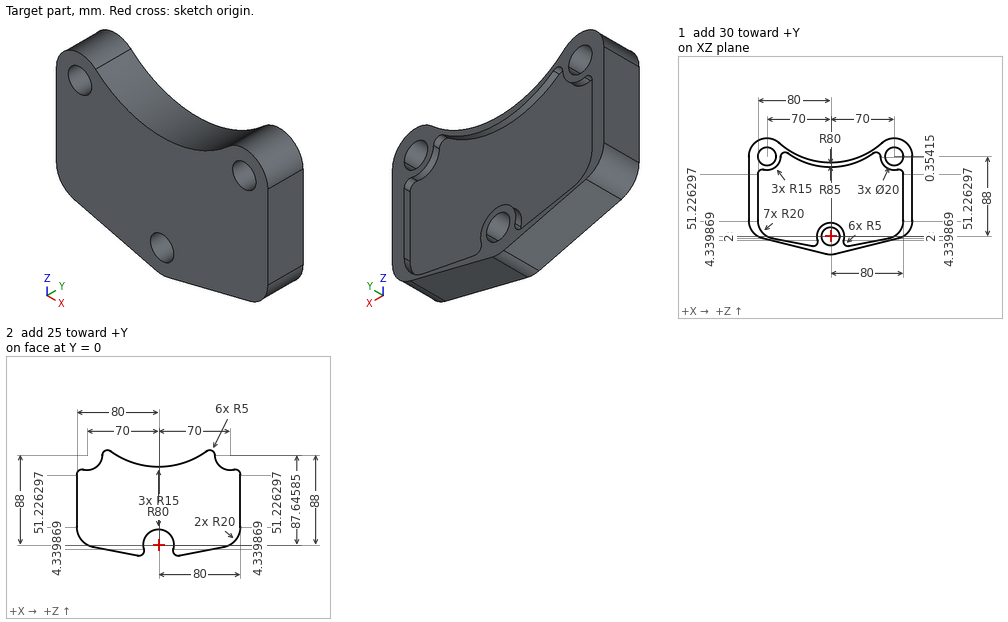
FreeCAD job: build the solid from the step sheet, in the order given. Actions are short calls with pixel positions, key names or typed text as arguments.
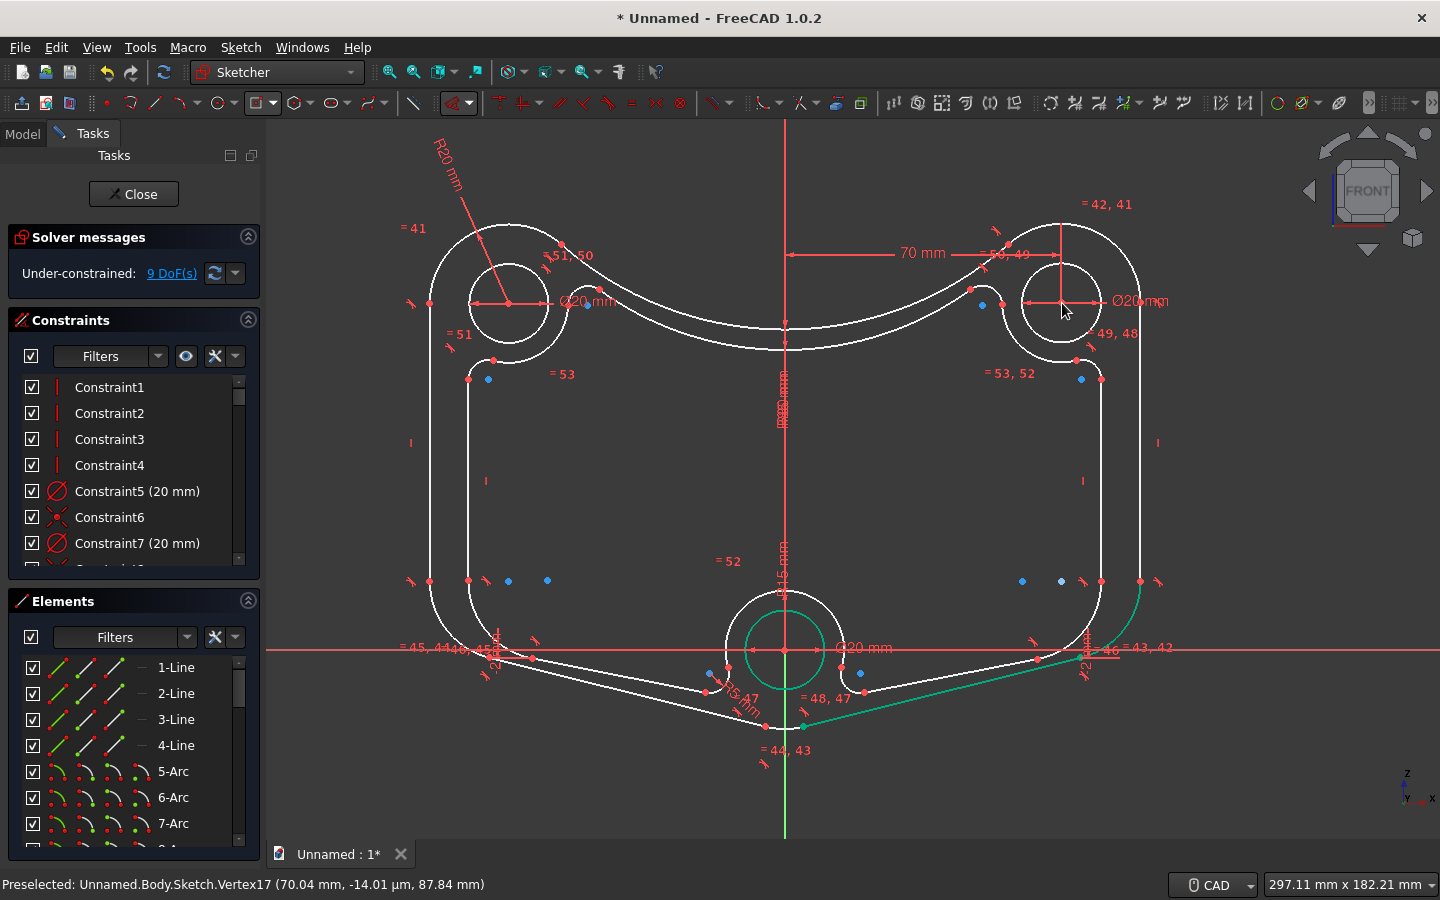
click(1061, 303)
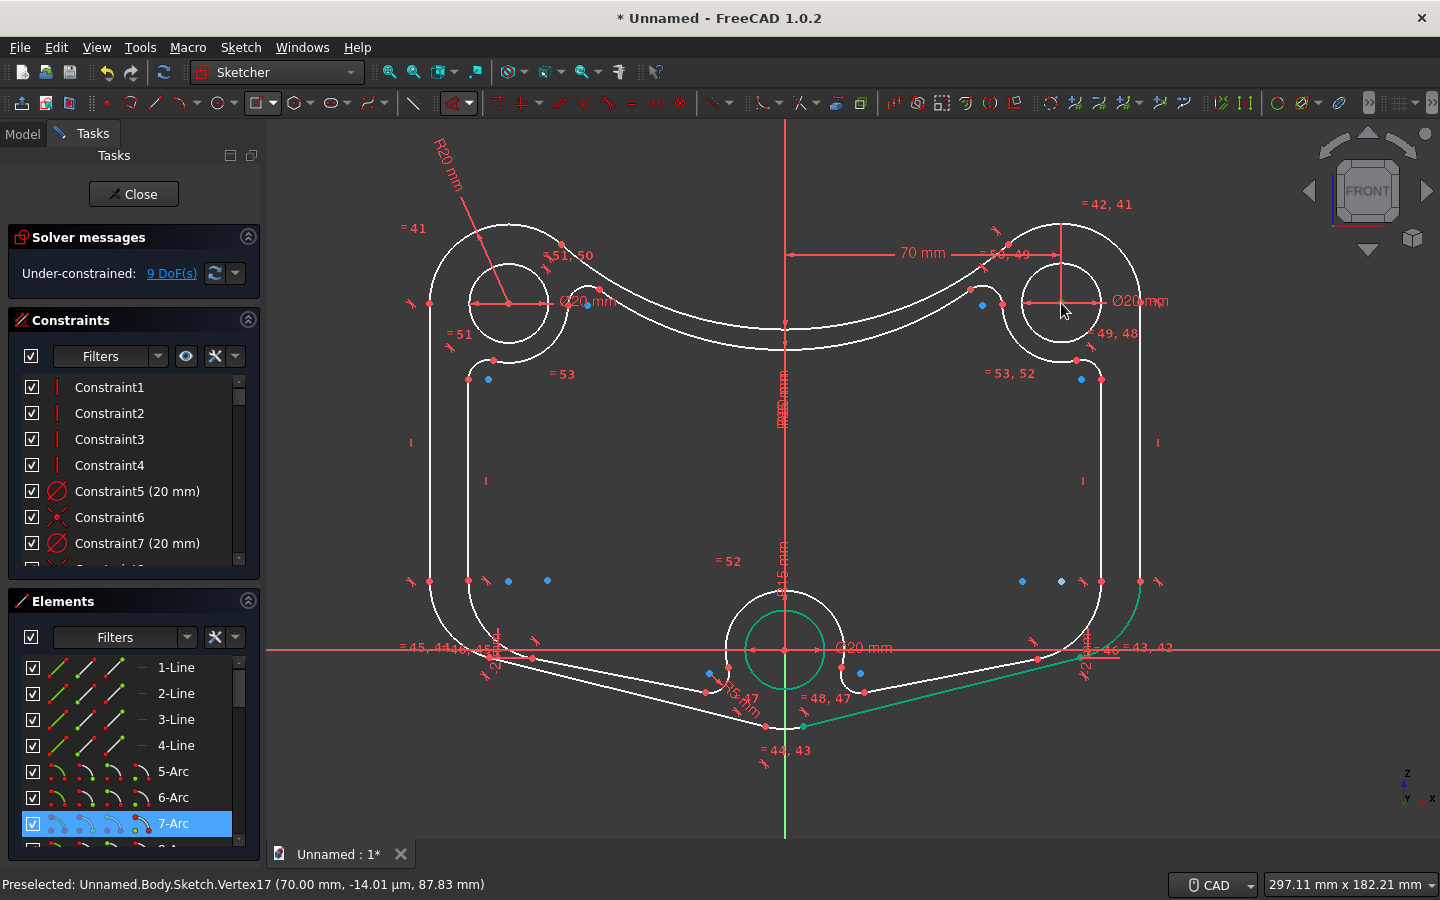
click(472, 104)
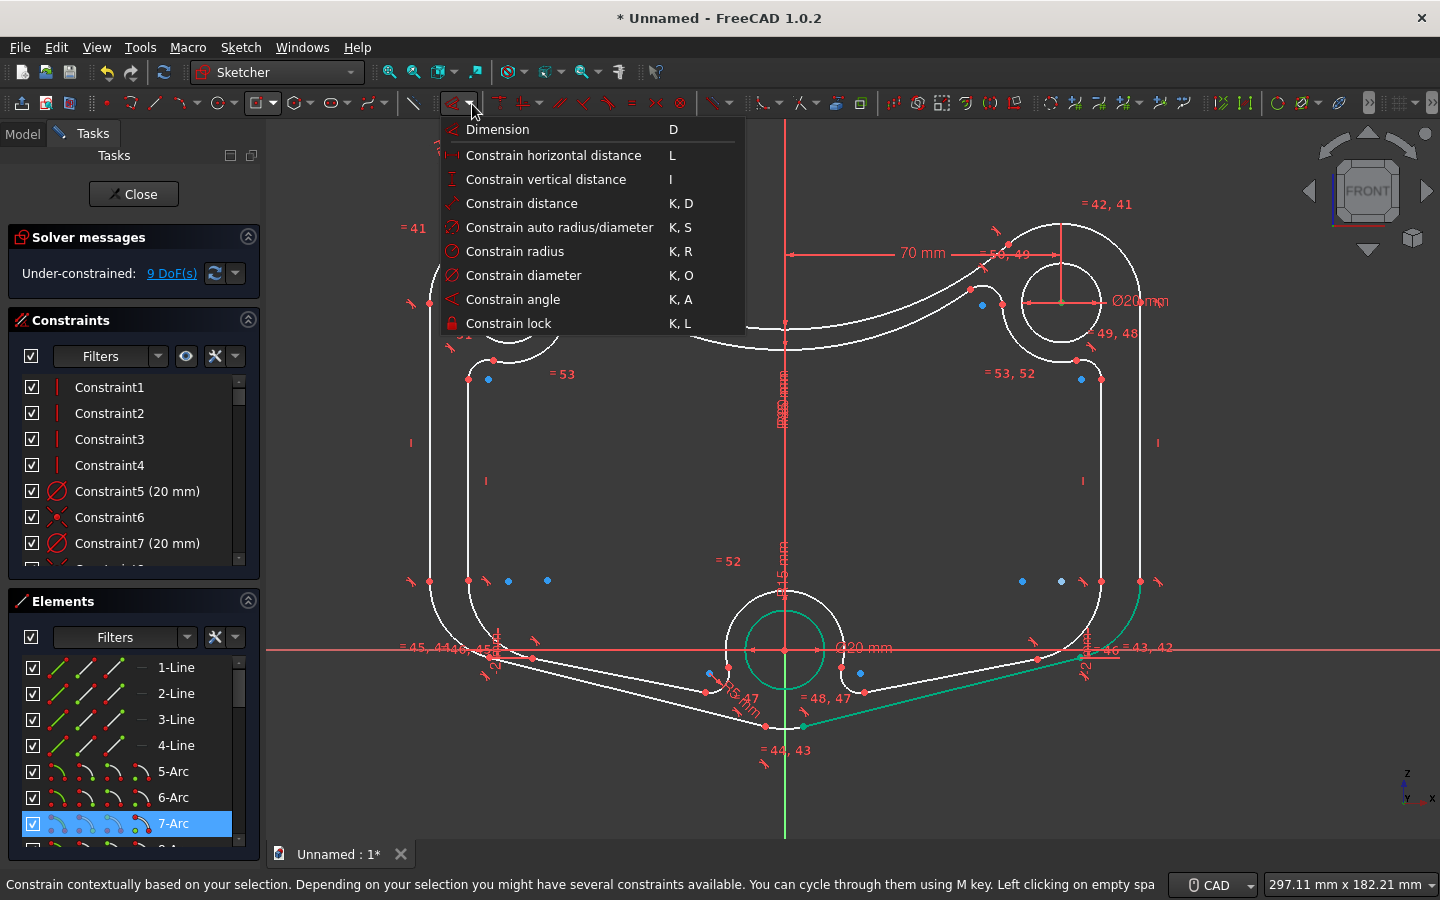
click(593, 179)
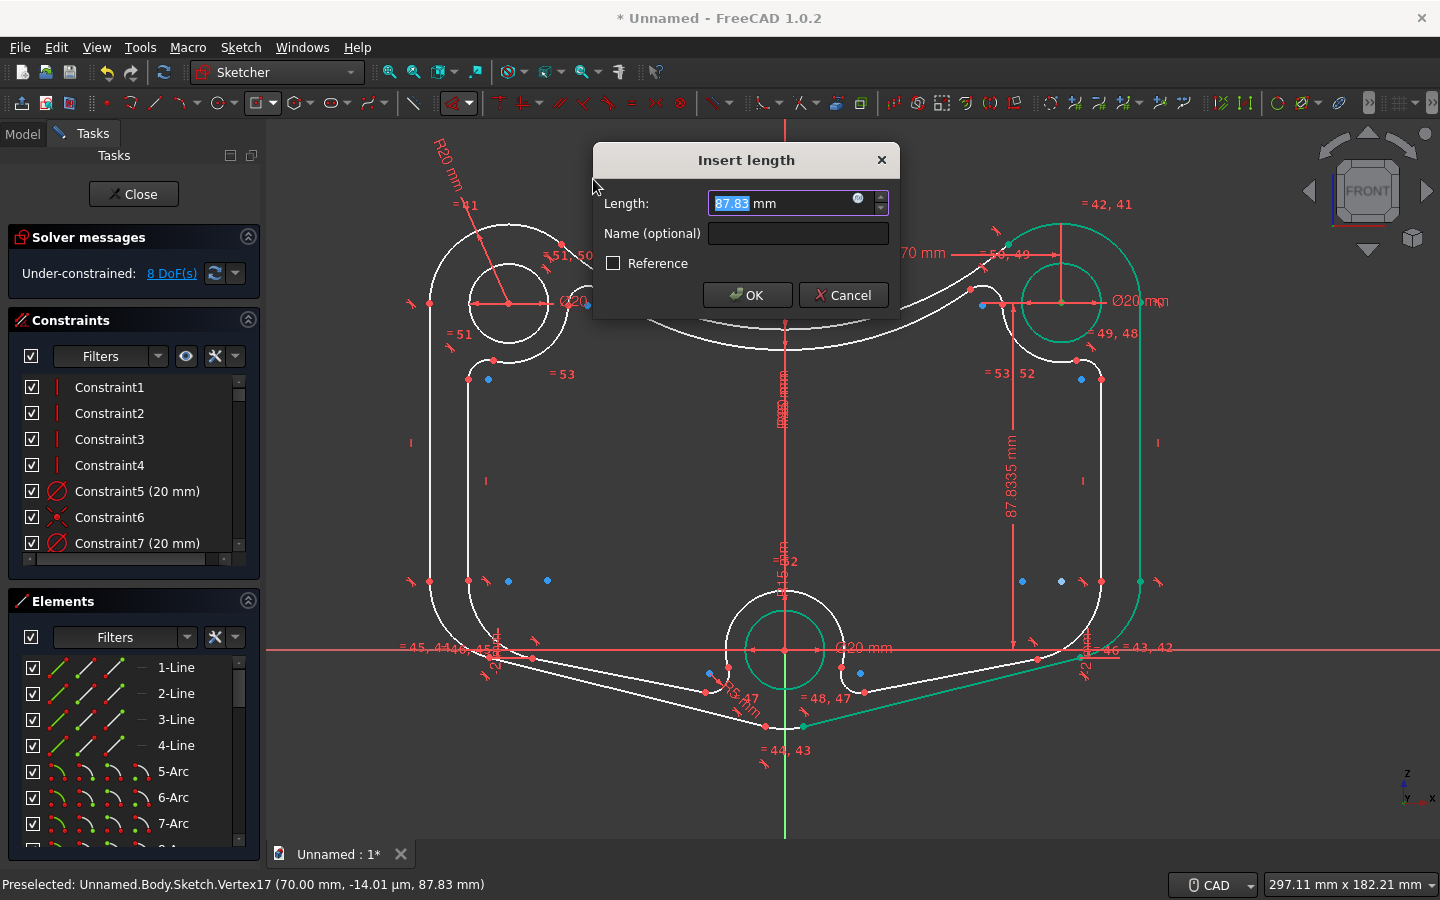
text(88)
key(Return)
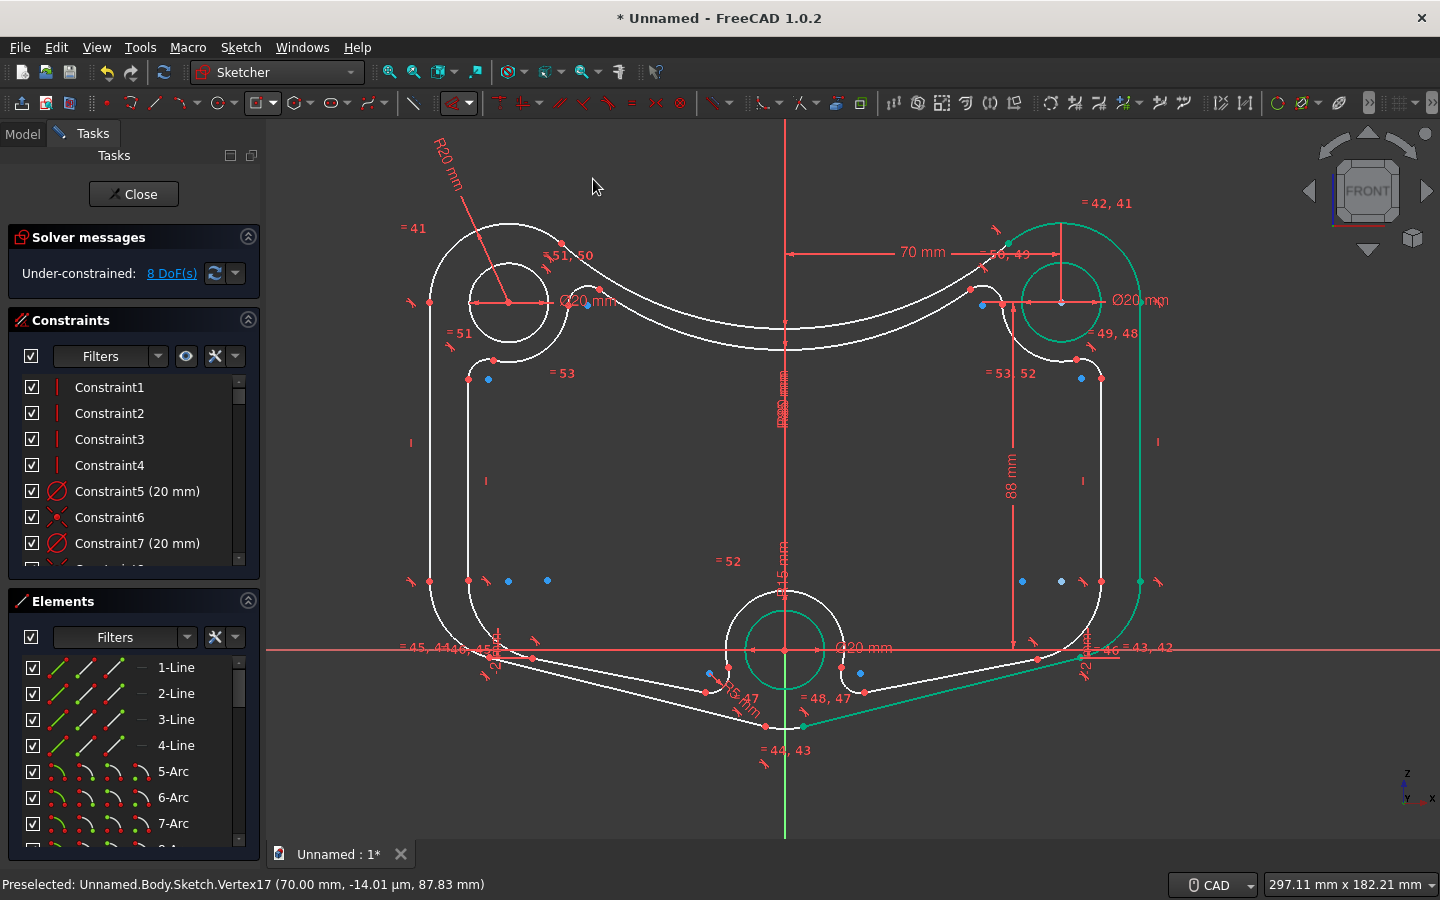
click(509, 303)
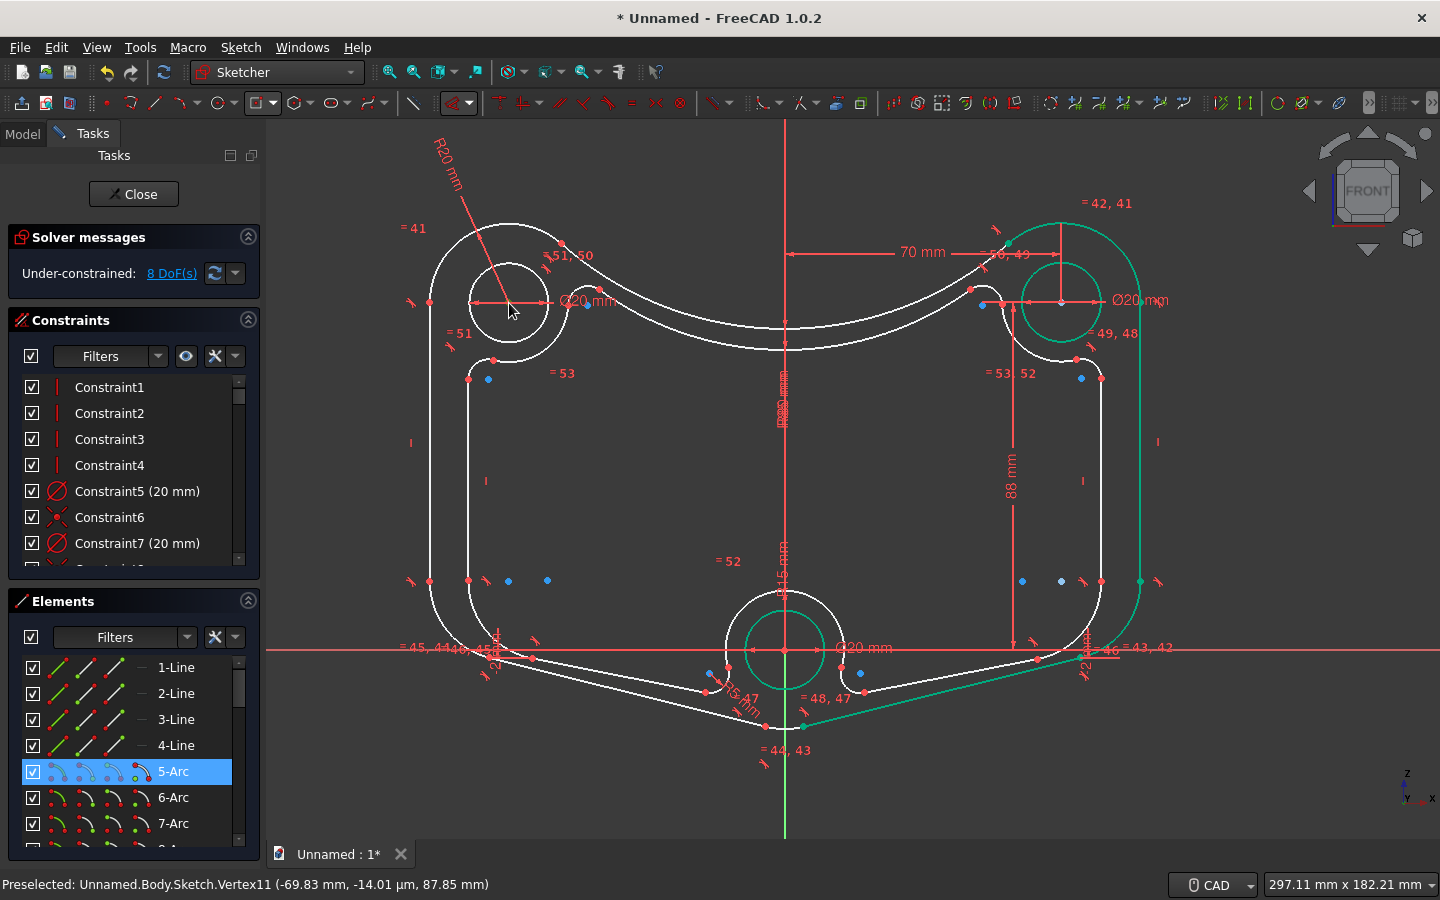
click(472, 104)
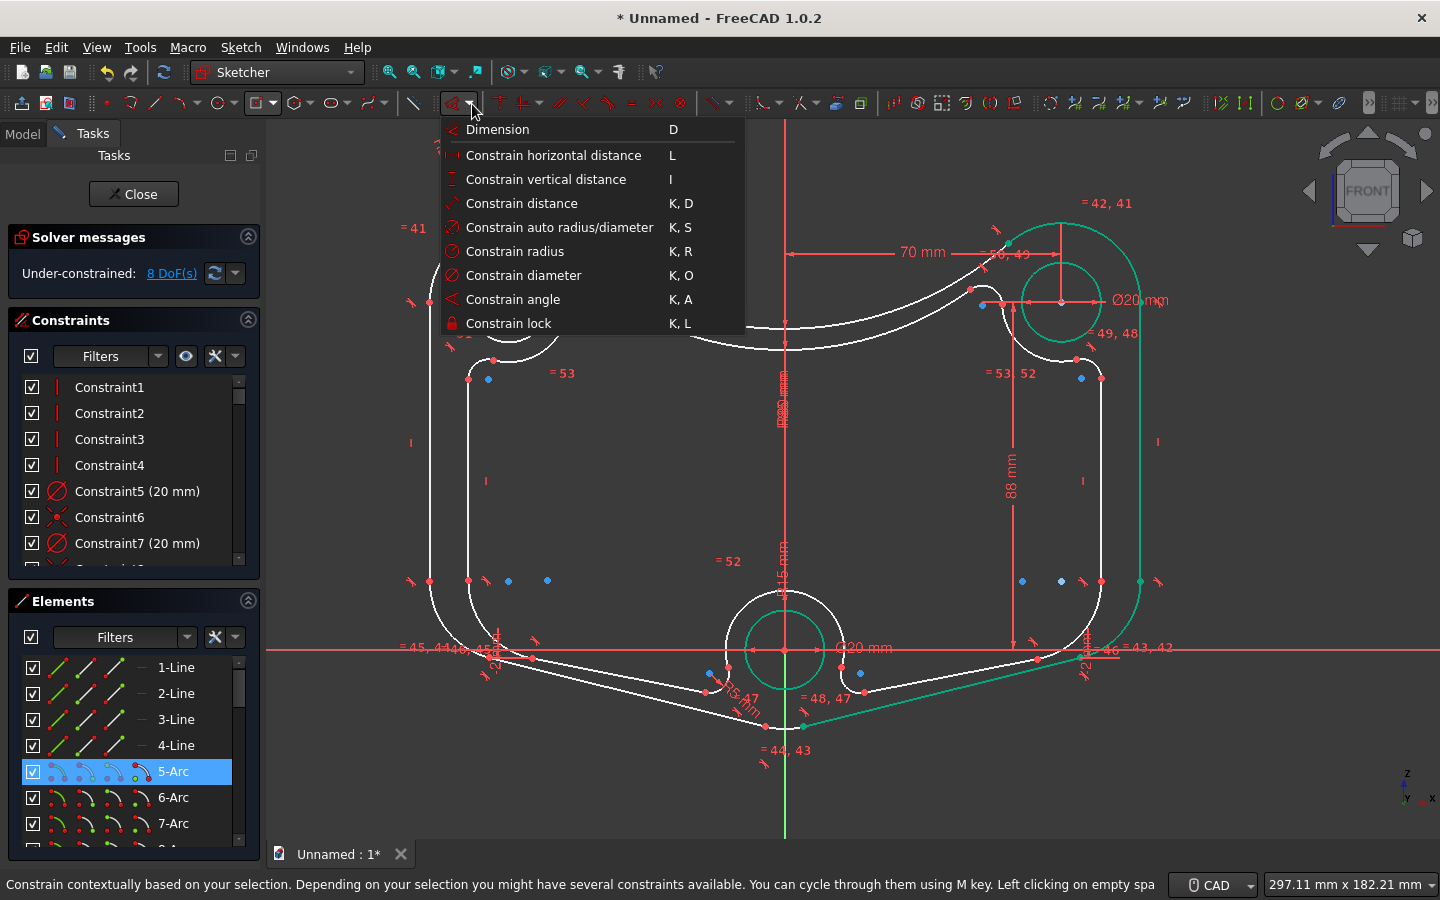
click(593, 155)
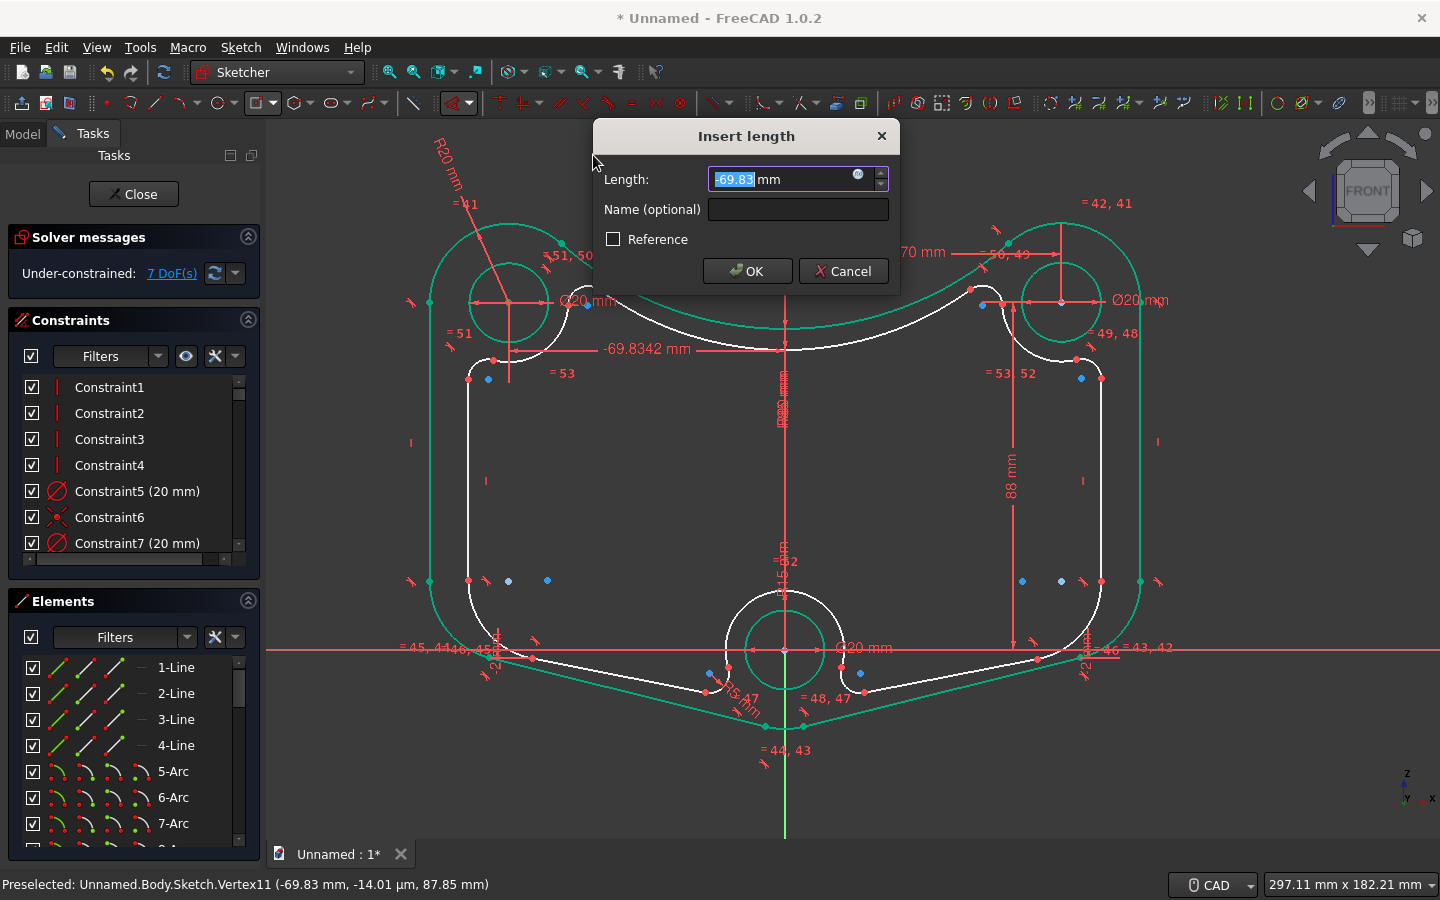
text(-70)
key(Return)